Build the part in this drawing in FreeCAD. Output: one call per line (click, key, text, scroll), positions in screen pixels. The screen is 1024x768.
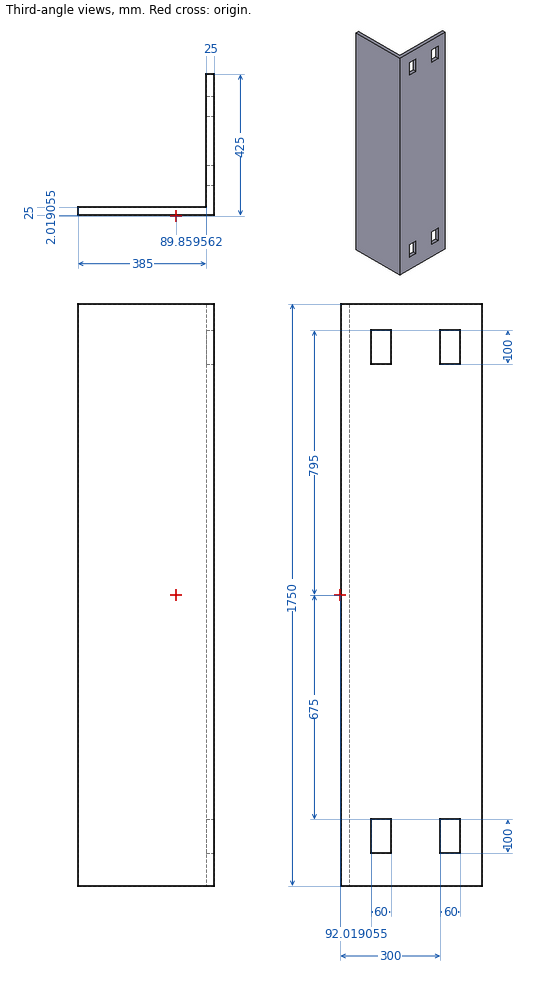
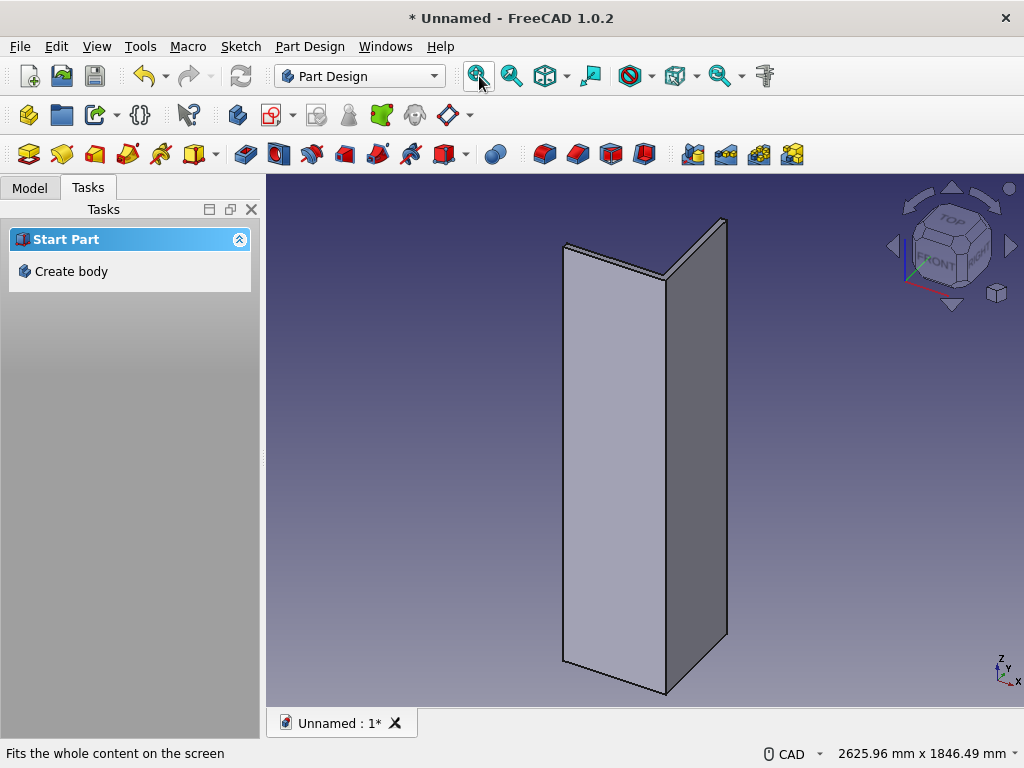
click(270, 116)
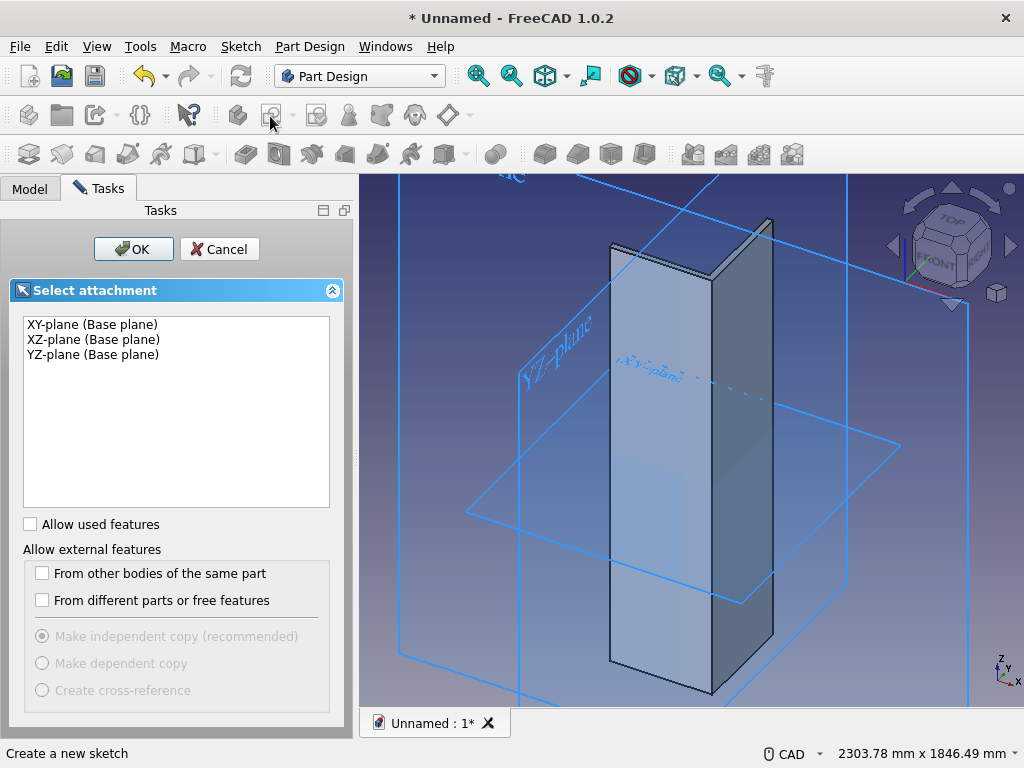
click(84, 354)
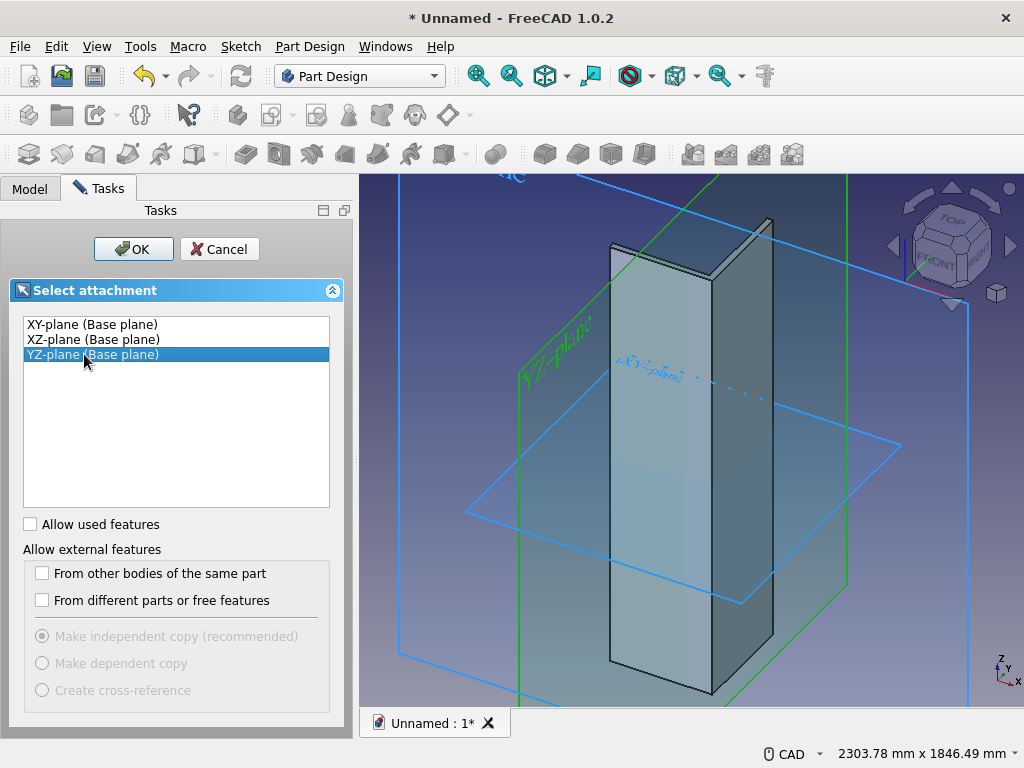
click(134, 249)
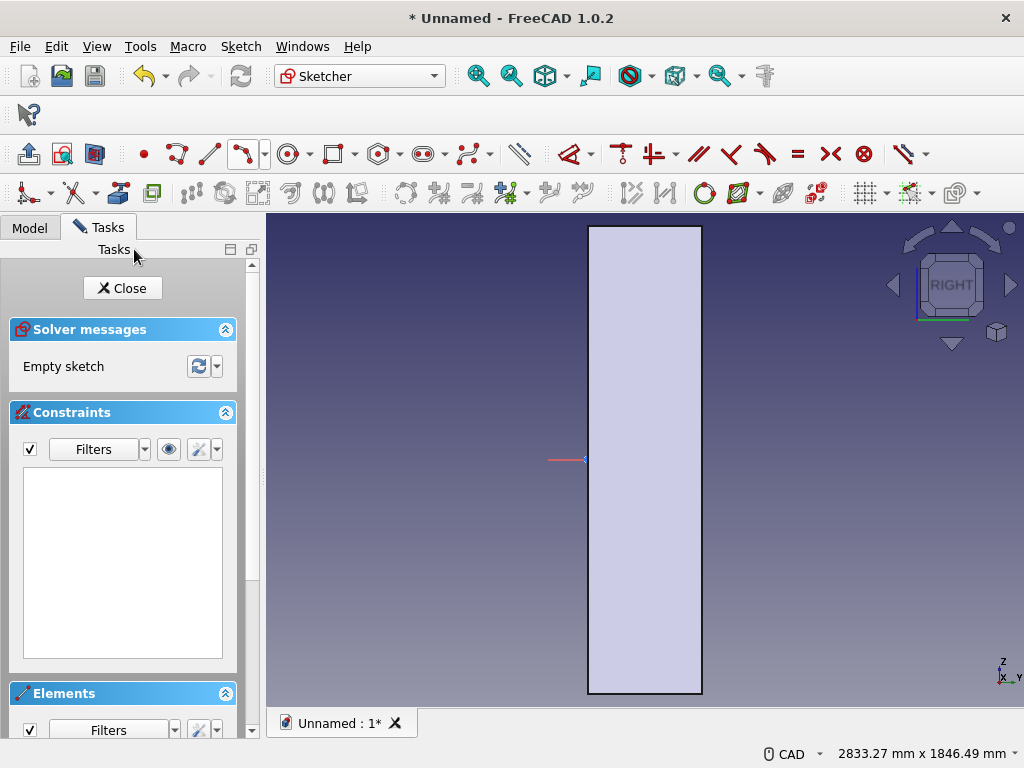
click(95, 154)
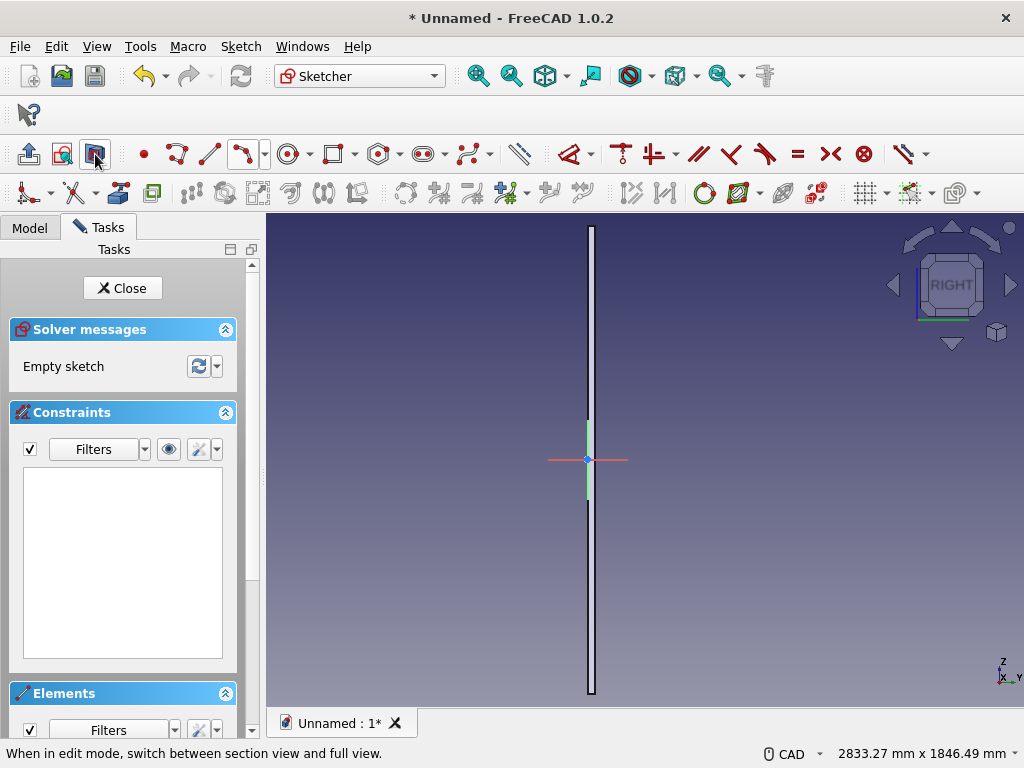
scroll(455, 465, down, 2)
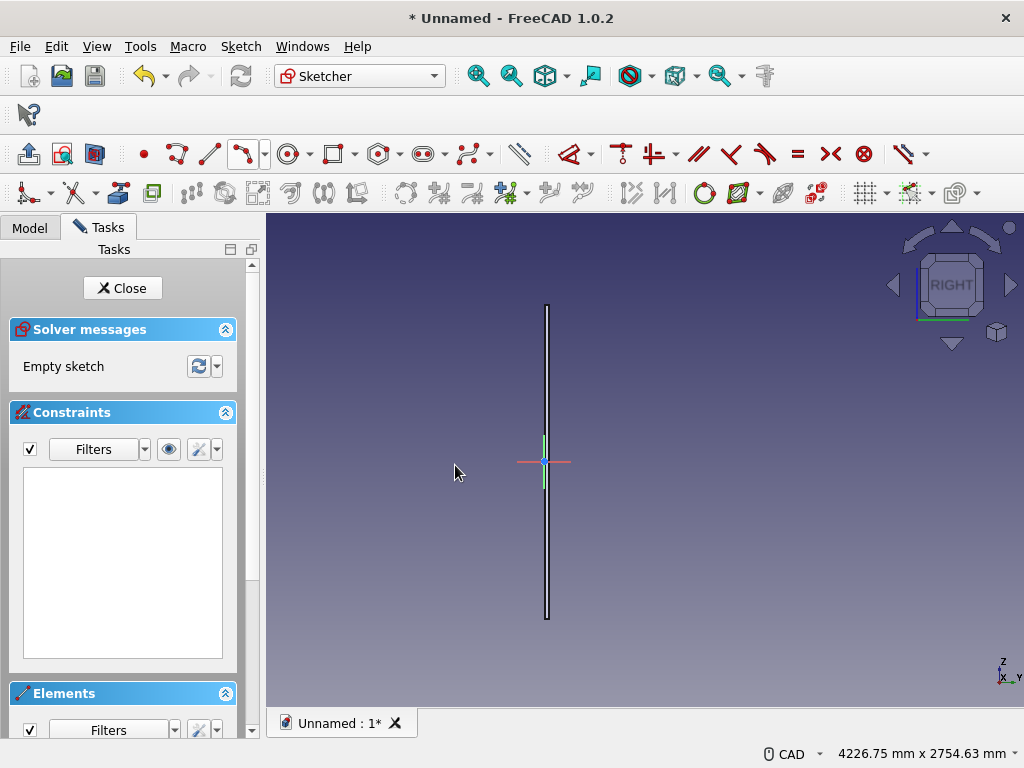
key(g)
key(r)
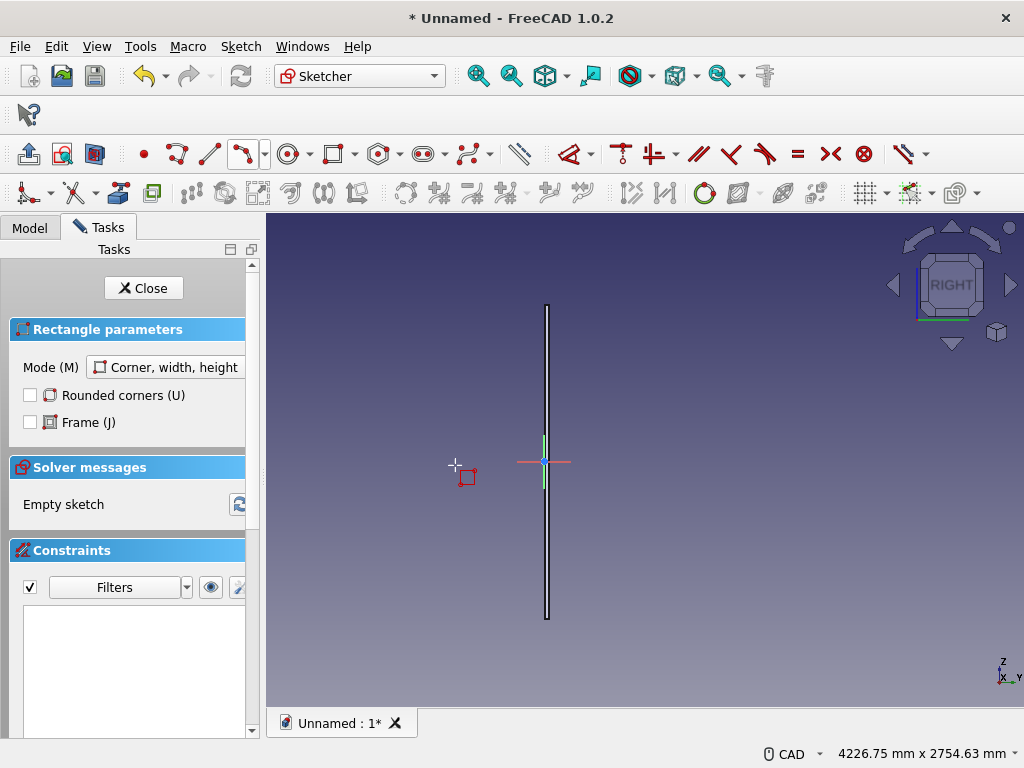
scroll(598, 583, up, 2)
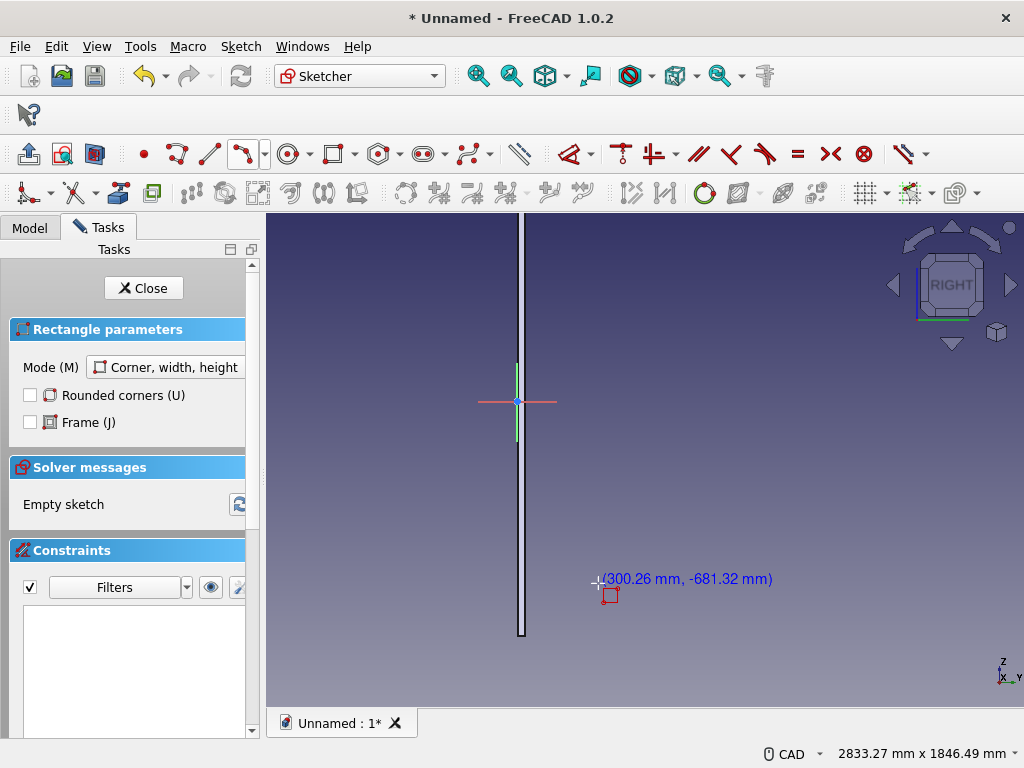
click(598, 582)
click(614, 609)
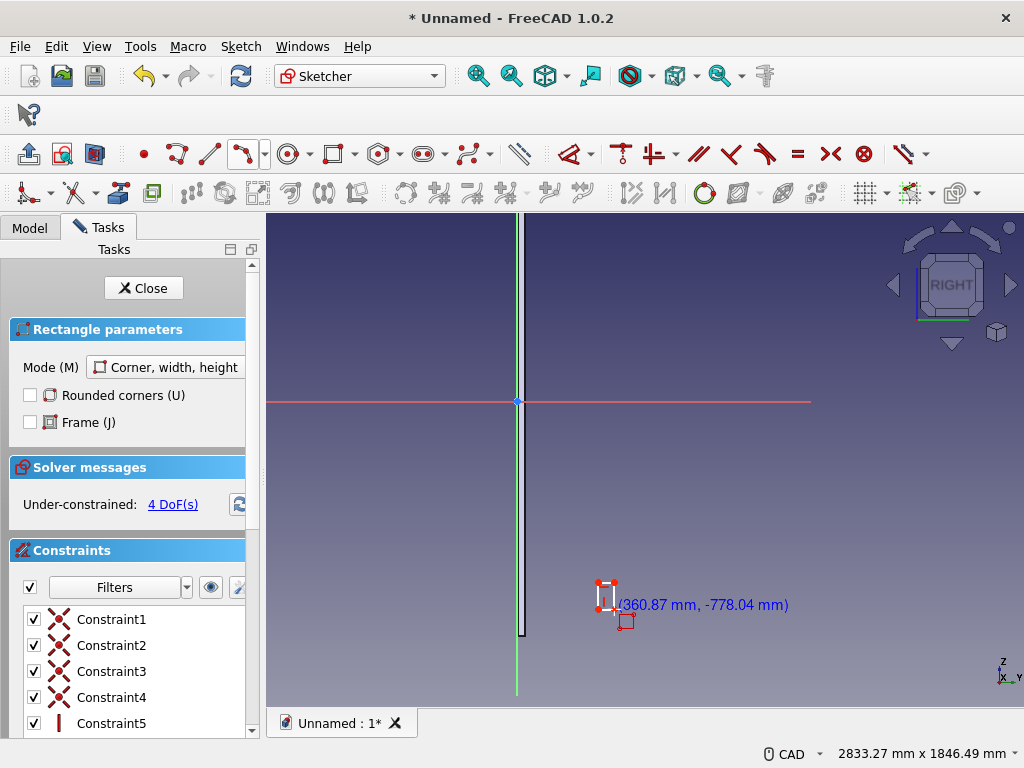
scroll(599, 584, down, 2)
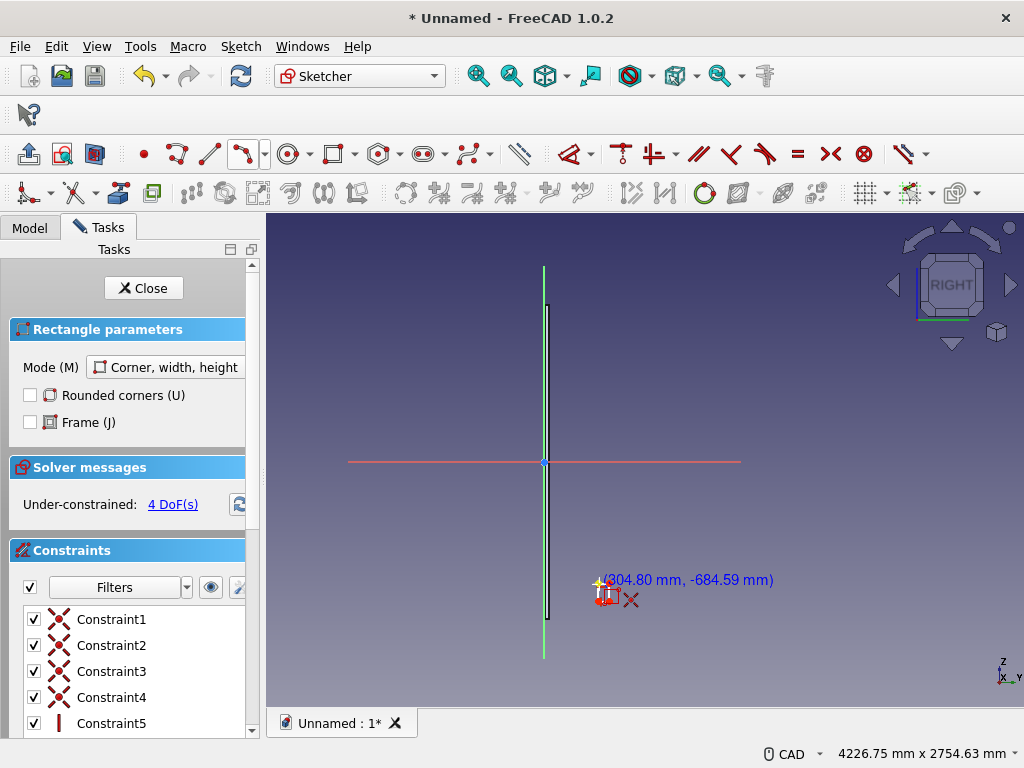
scroll(598, 320, up, 2)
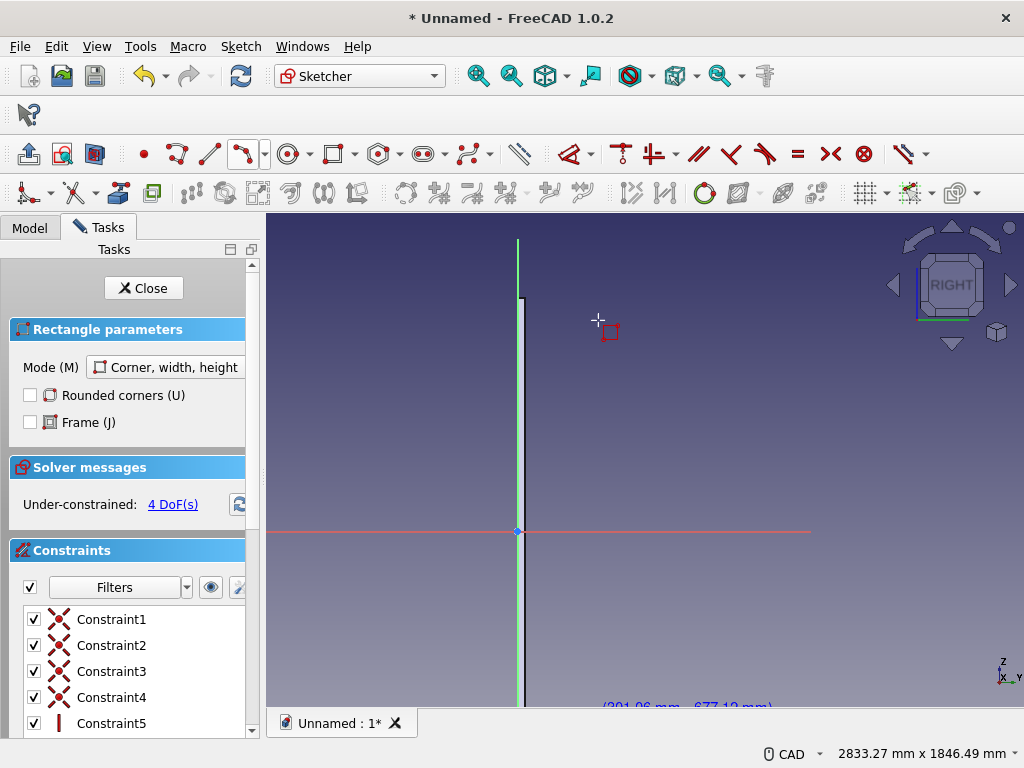
click(598, 319)
click(614, 346)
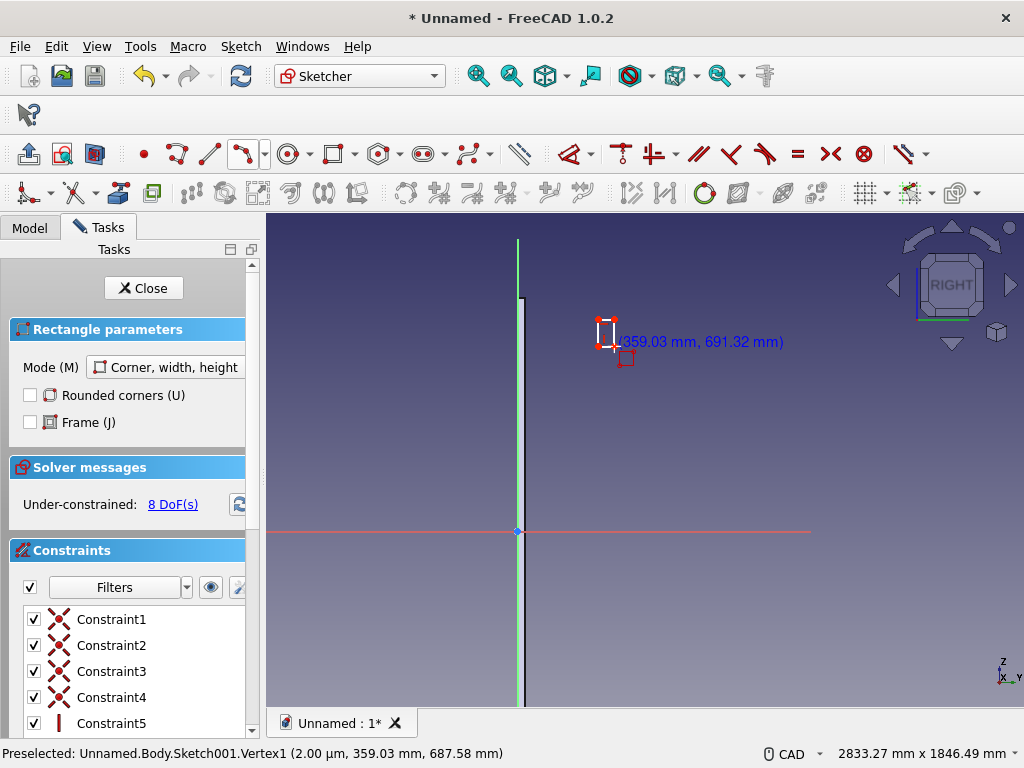
scroll(598, 319, down, 2)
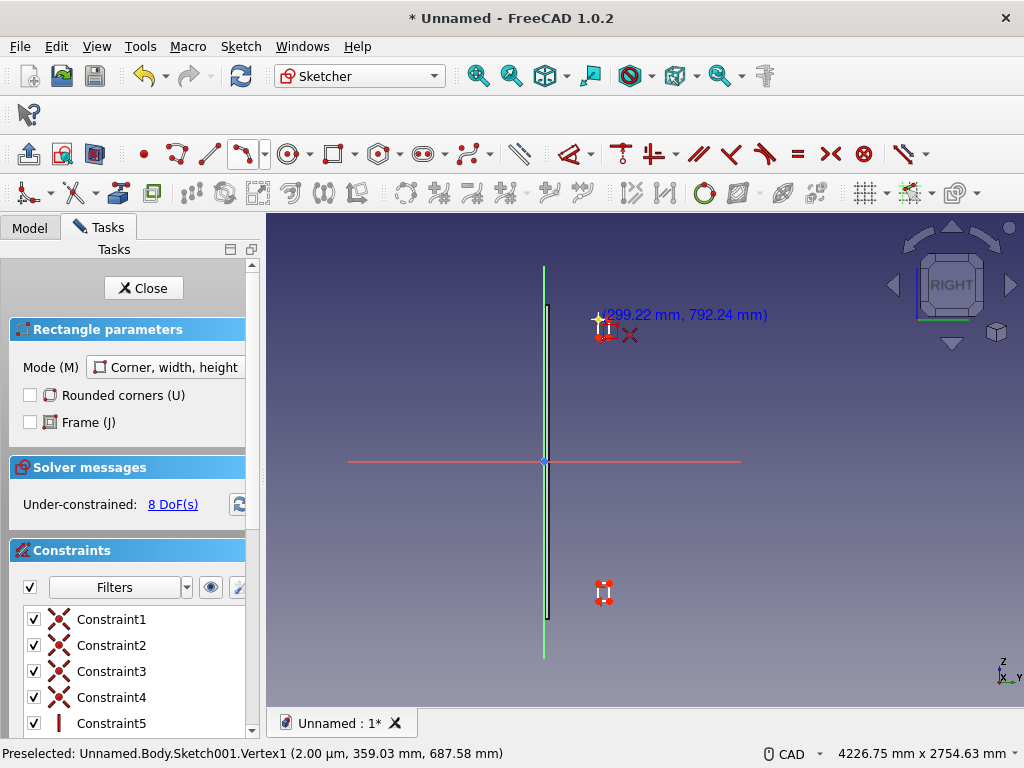
scroll(561, 583, up, 2)